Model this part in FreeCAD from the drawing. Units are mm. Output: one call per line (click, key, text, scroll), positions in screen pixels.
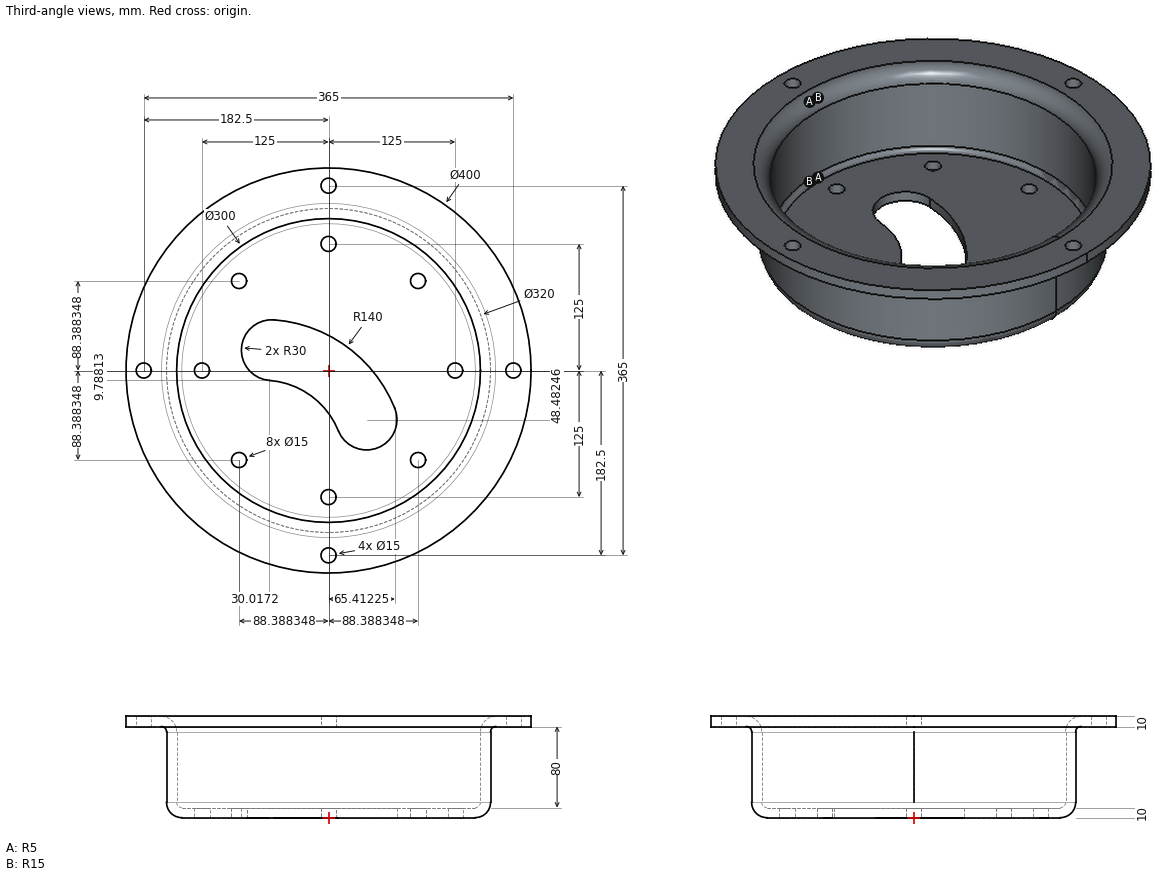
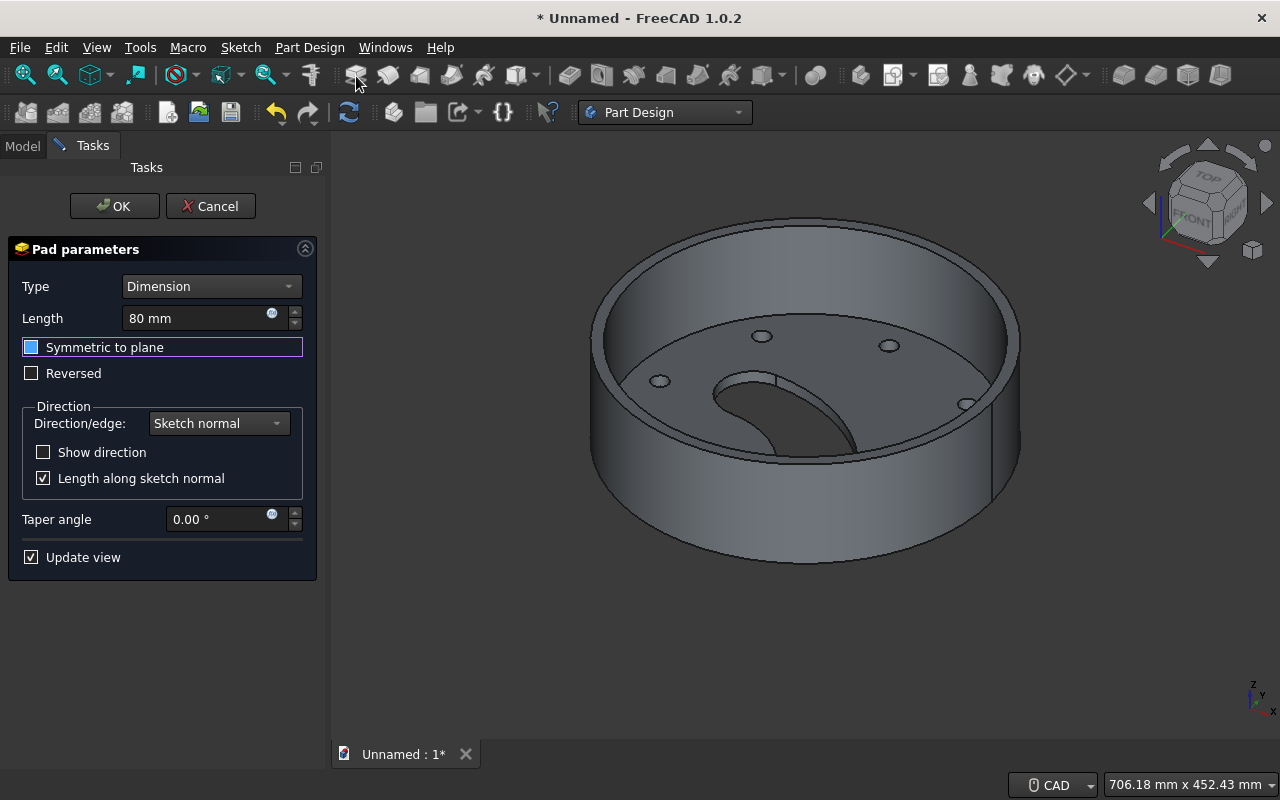
click(115, 206)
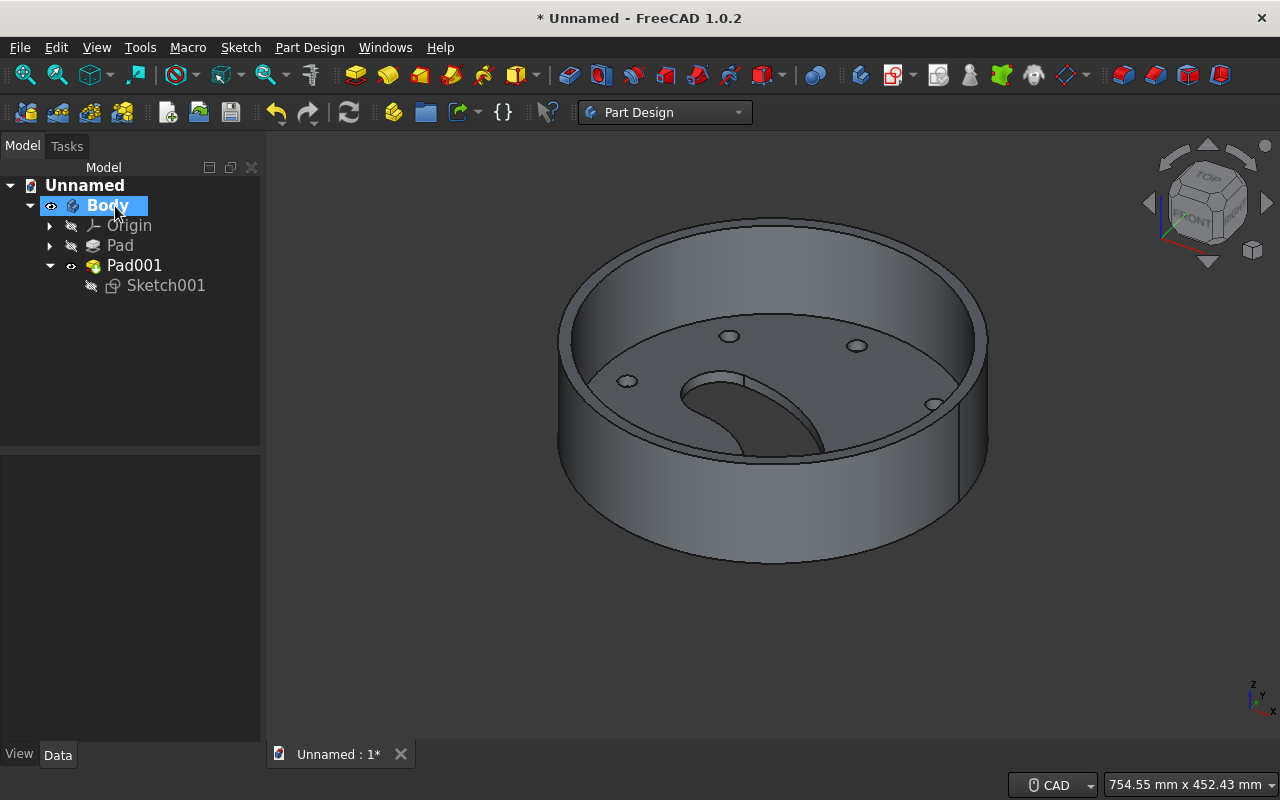
scroll(838, 226, up, 5)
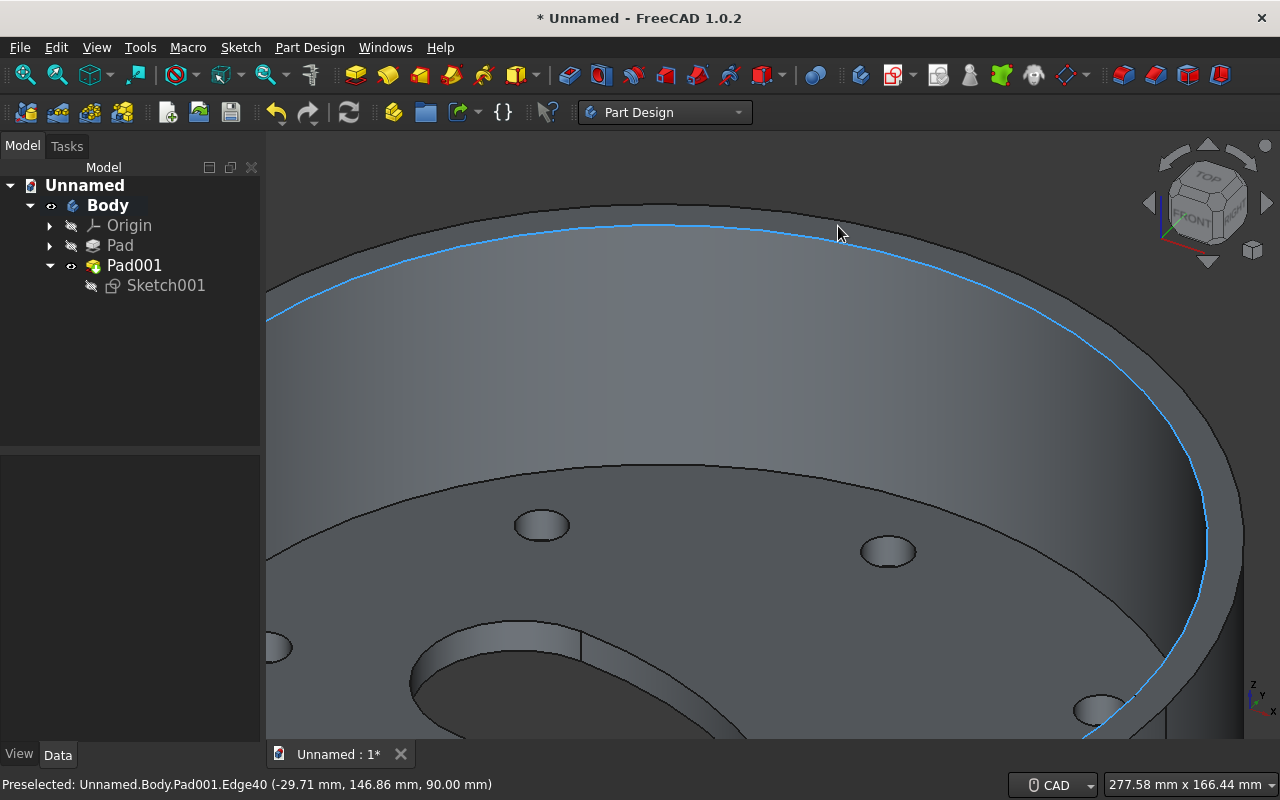
click(838, 226)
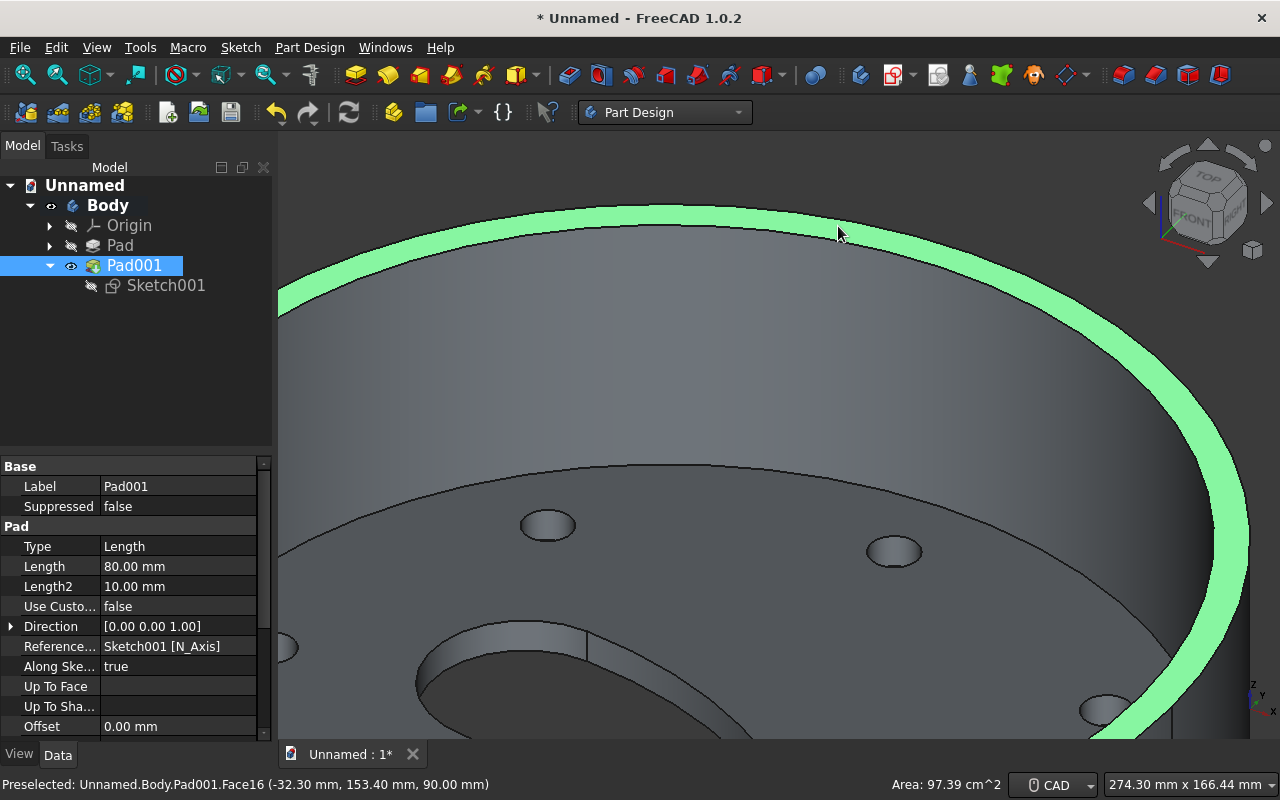
click(894, 76)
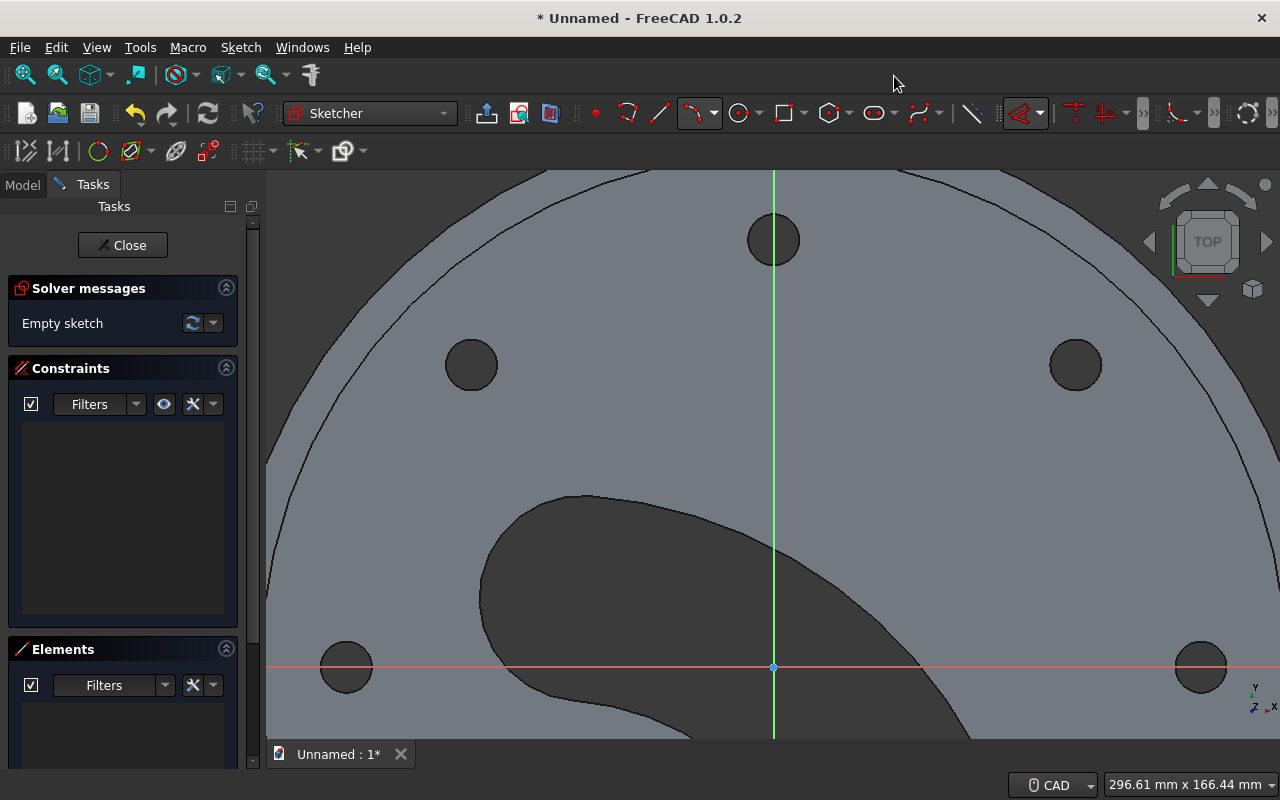
scroll(682, 385, down, 7)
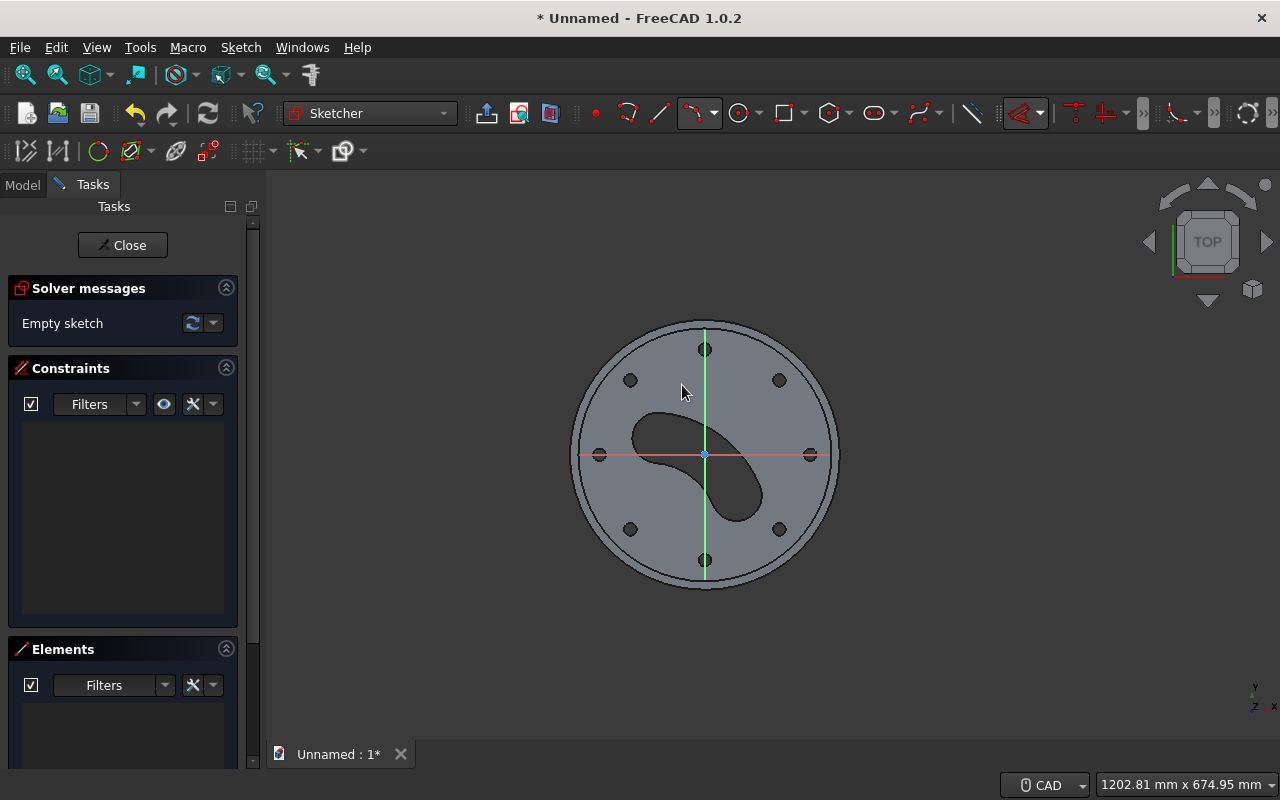
click(740, 114)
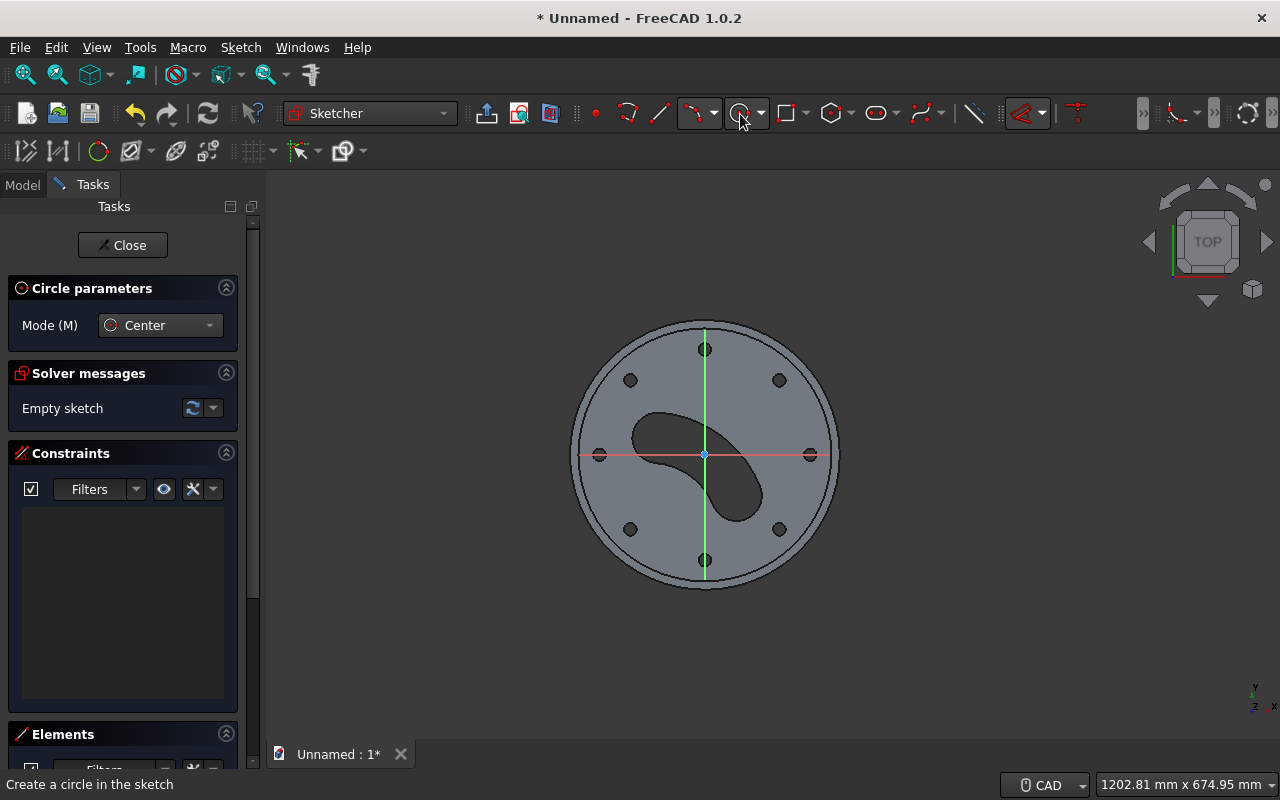
click(705, 455)
click(824, 336)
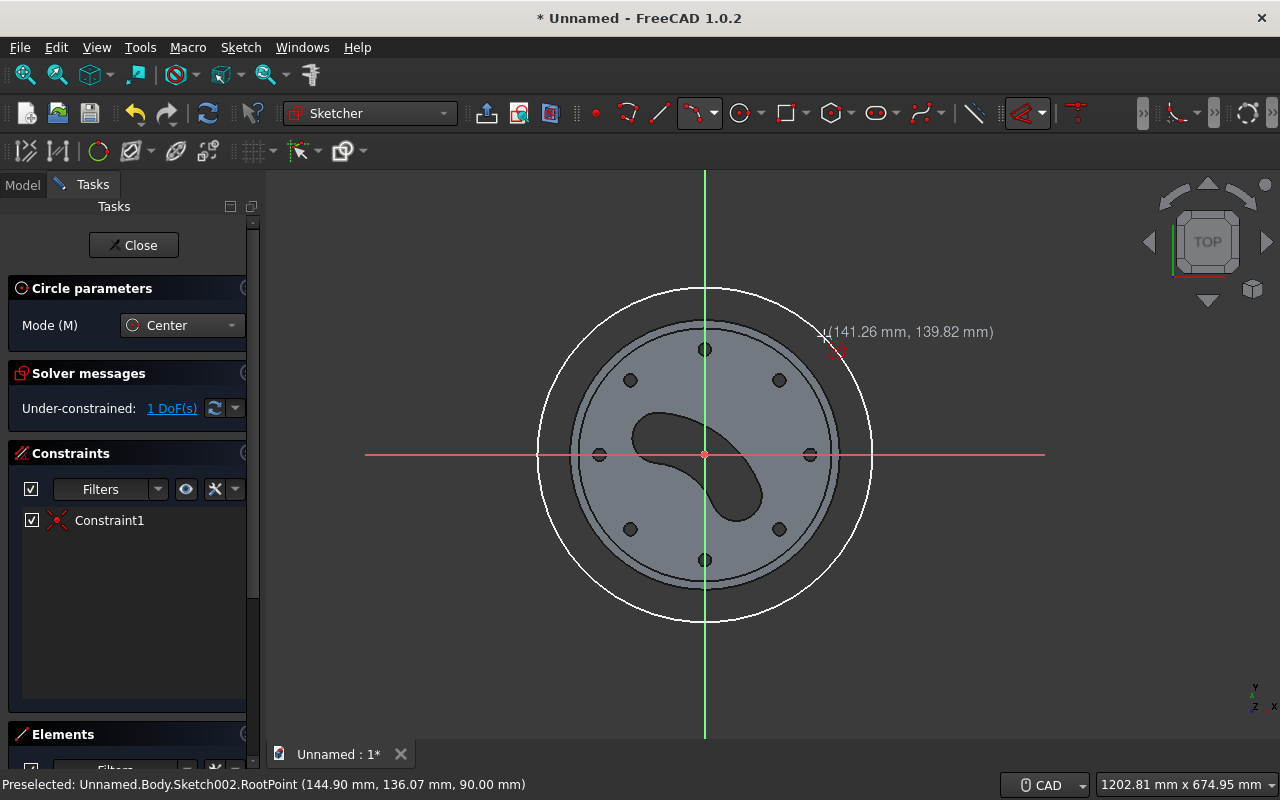
scroll(705, 609, up, 7)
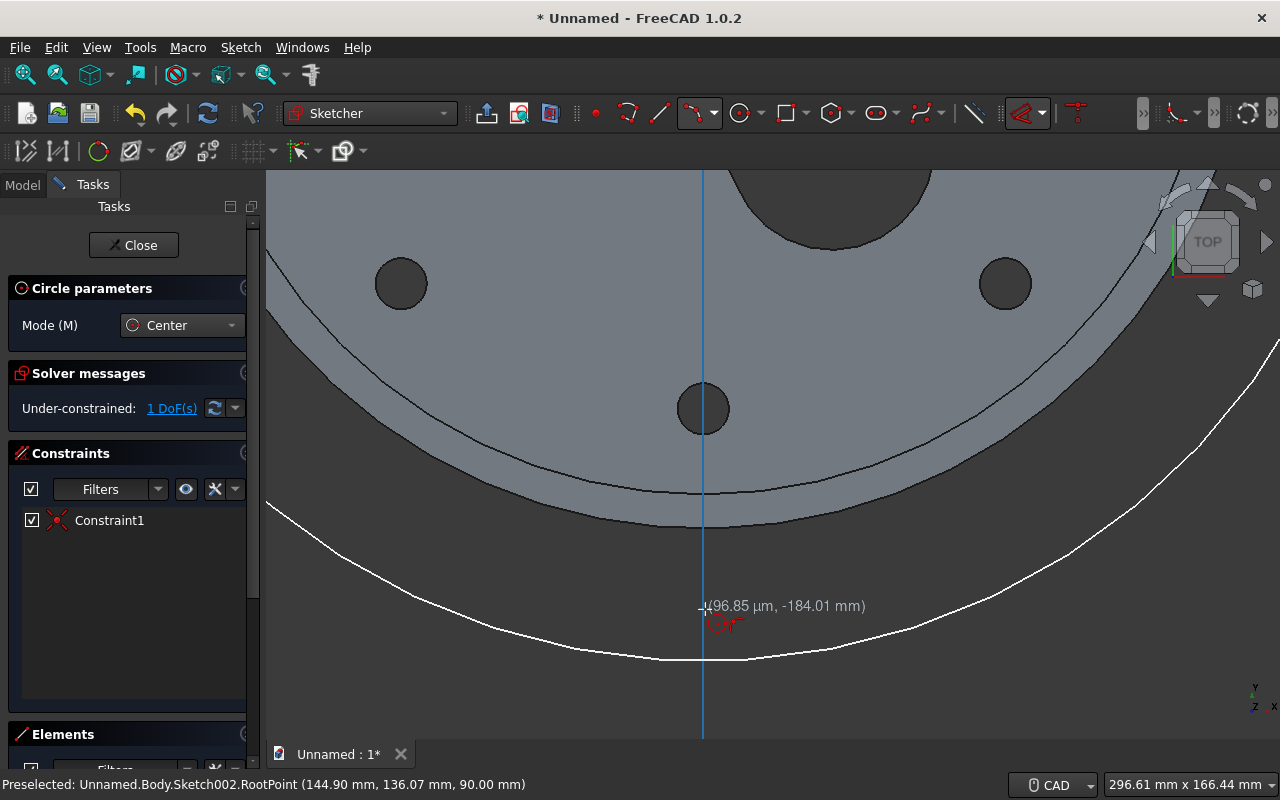
scroll(705, 609, down, 7)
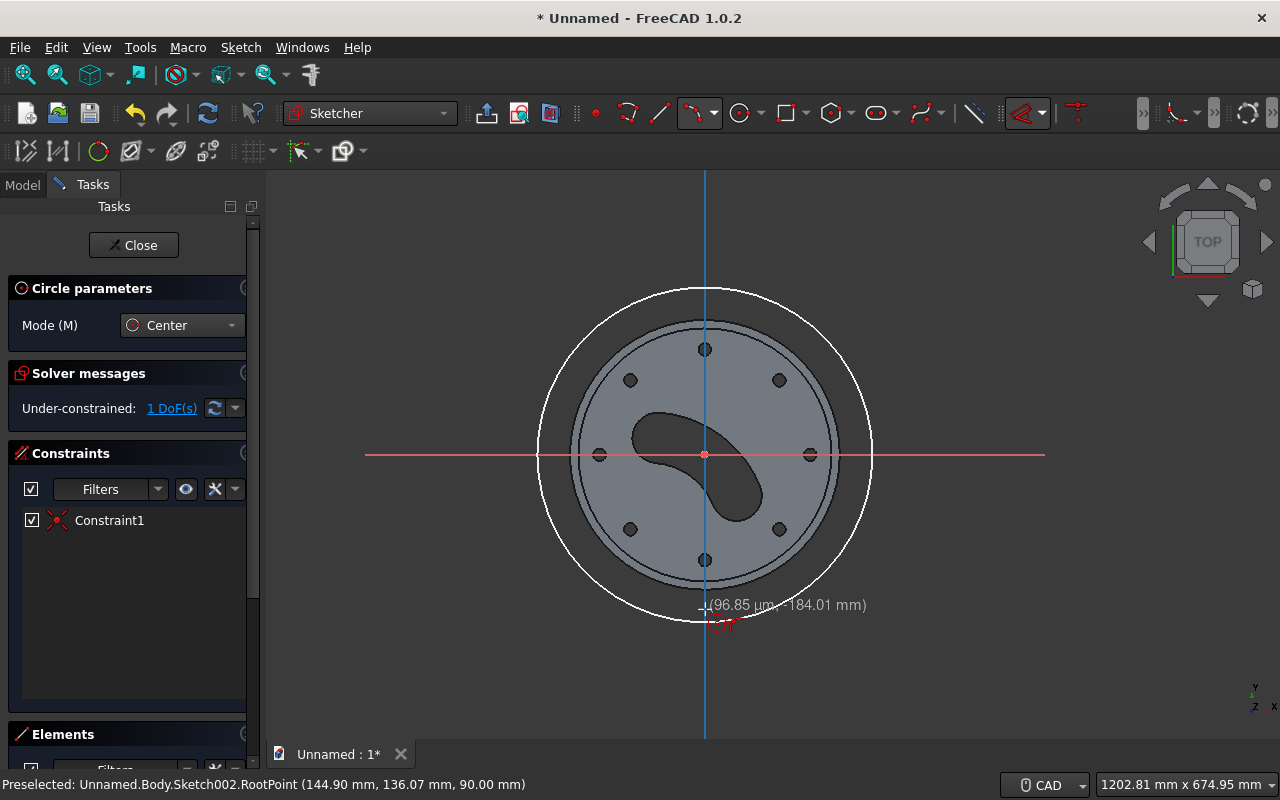
click(705, 609)